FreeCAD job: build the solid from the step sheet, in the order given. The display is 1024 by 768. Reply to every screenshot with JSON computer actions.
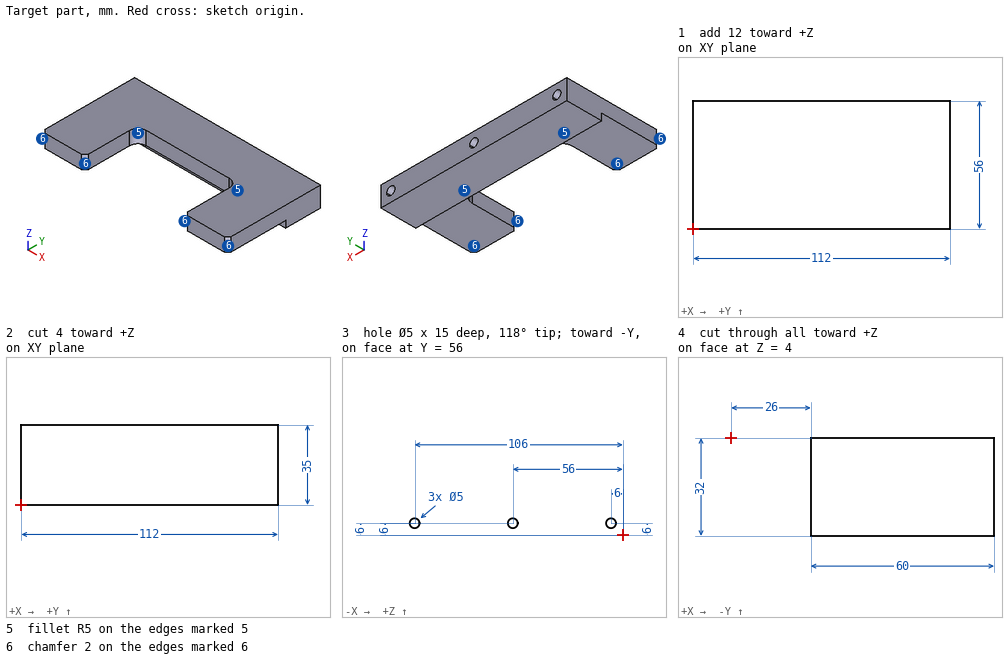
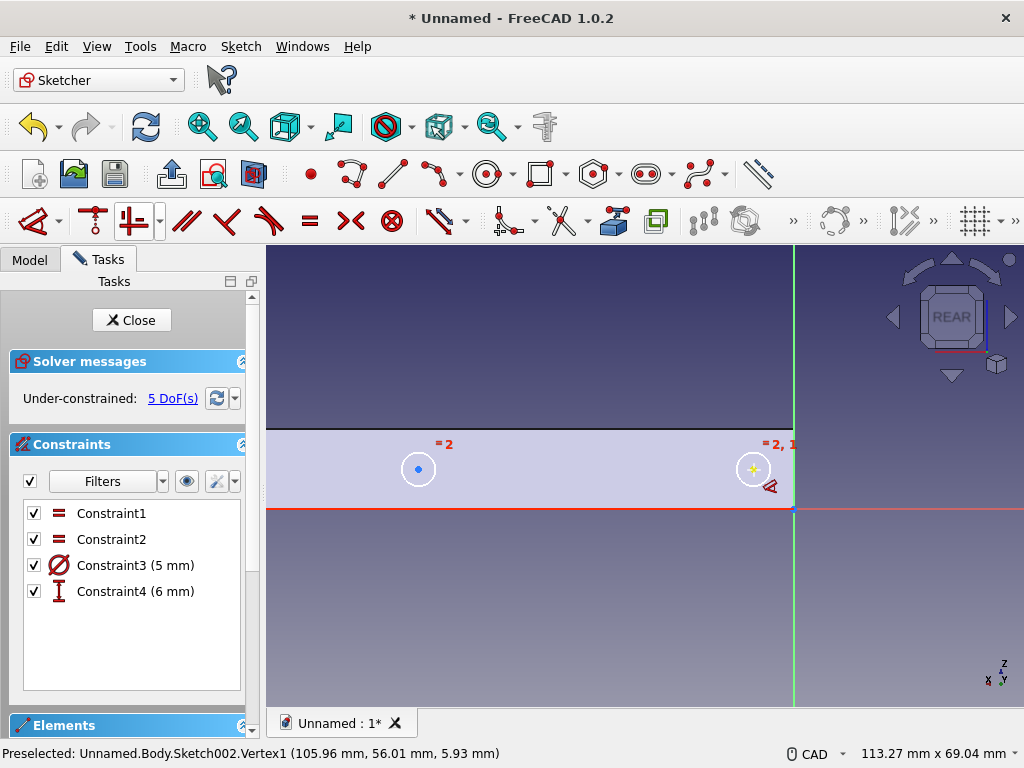
{"action": "left_click", "coordinate": [754, 469]}
{"action": "left_click", "coordinate": [774, 543]}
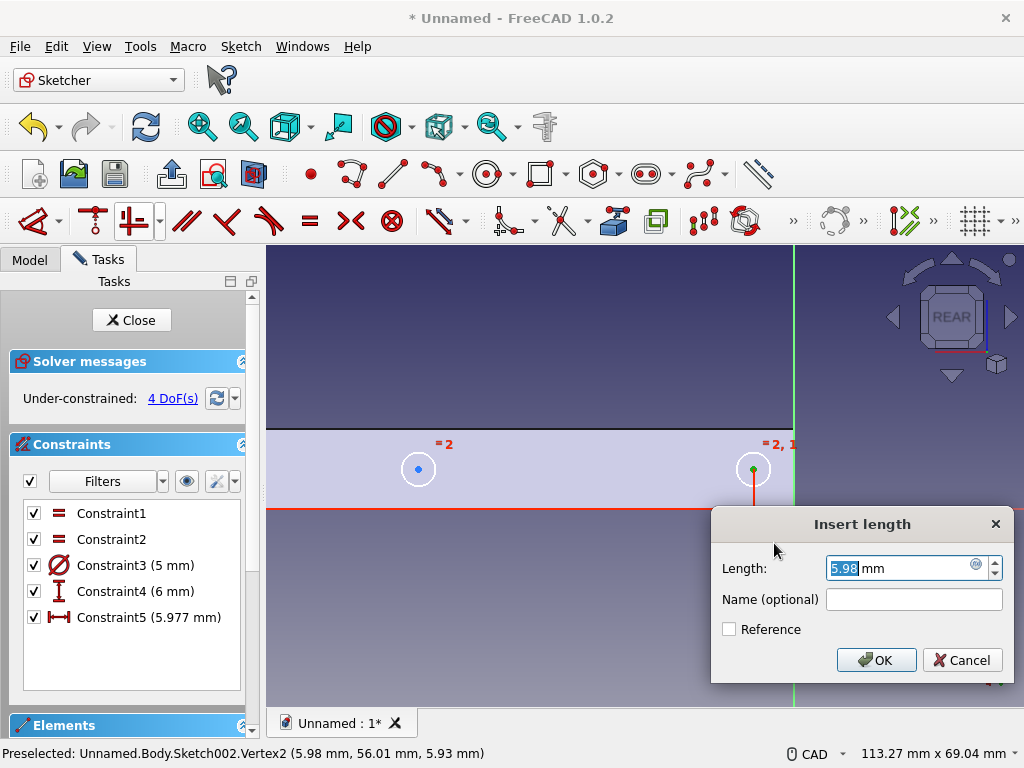
{"action": "type", "text": "6"}
{"action": "key", "text": "Return"}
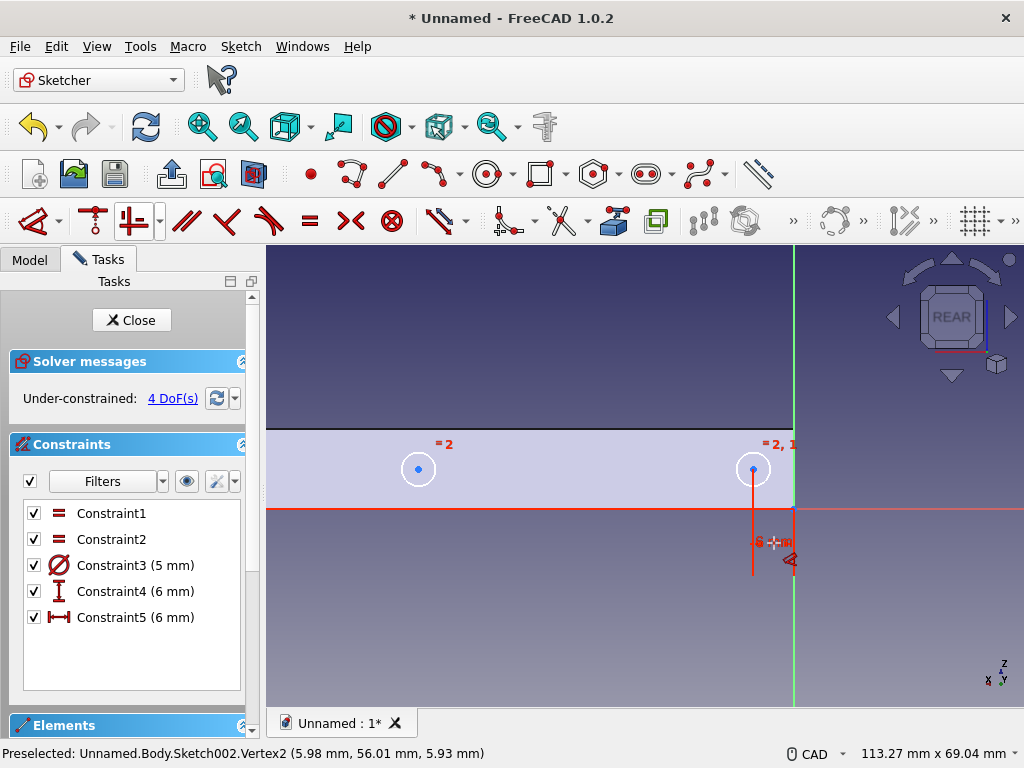
{"action": "left_click", "coordinate": [753, 469]}
{"action": "left_click", "coordinate": [828, 489]}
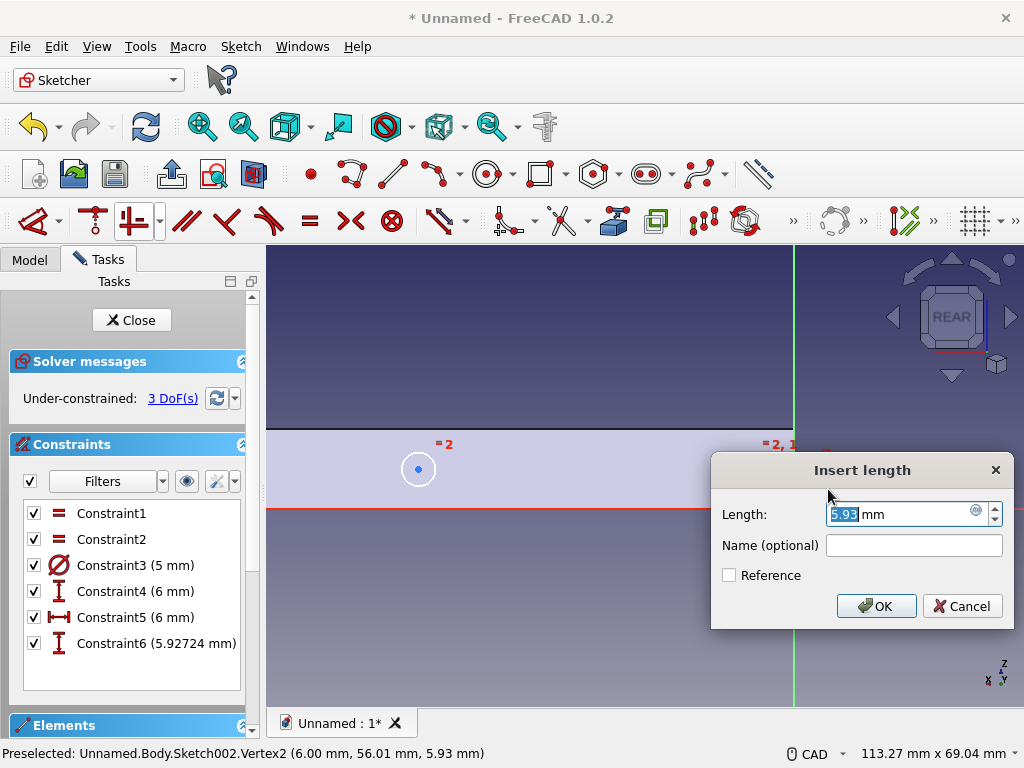
{"action": "type", "text": "6"}
{"action": "key", "text": "Return"}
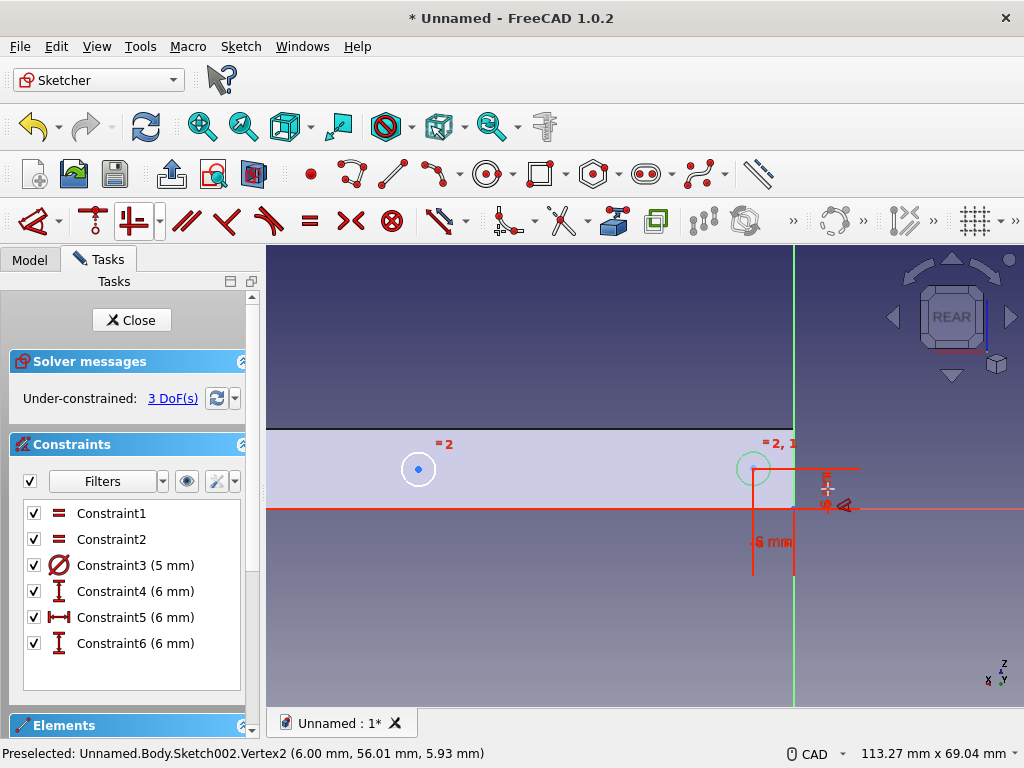
{"action": "left_click", "coordinate": [419, 469]}
{"action": "left_click", "coordinate": [385, 489]}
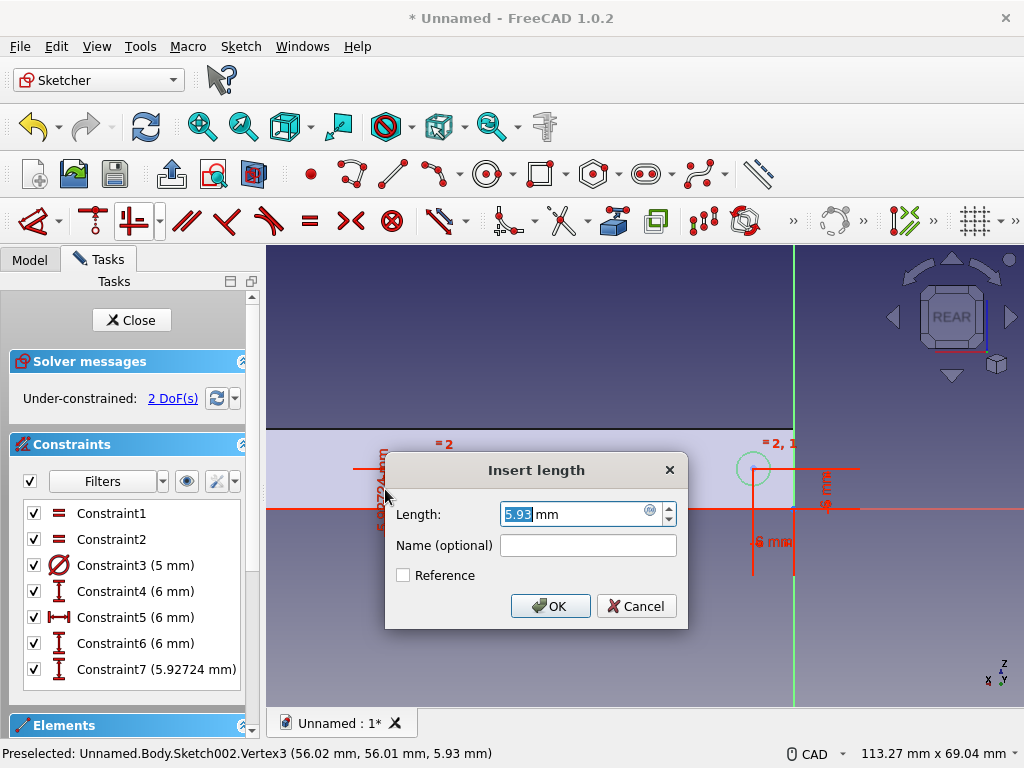
{"action": "type", "text": "6"}
{"action": "key", "text": "Return"}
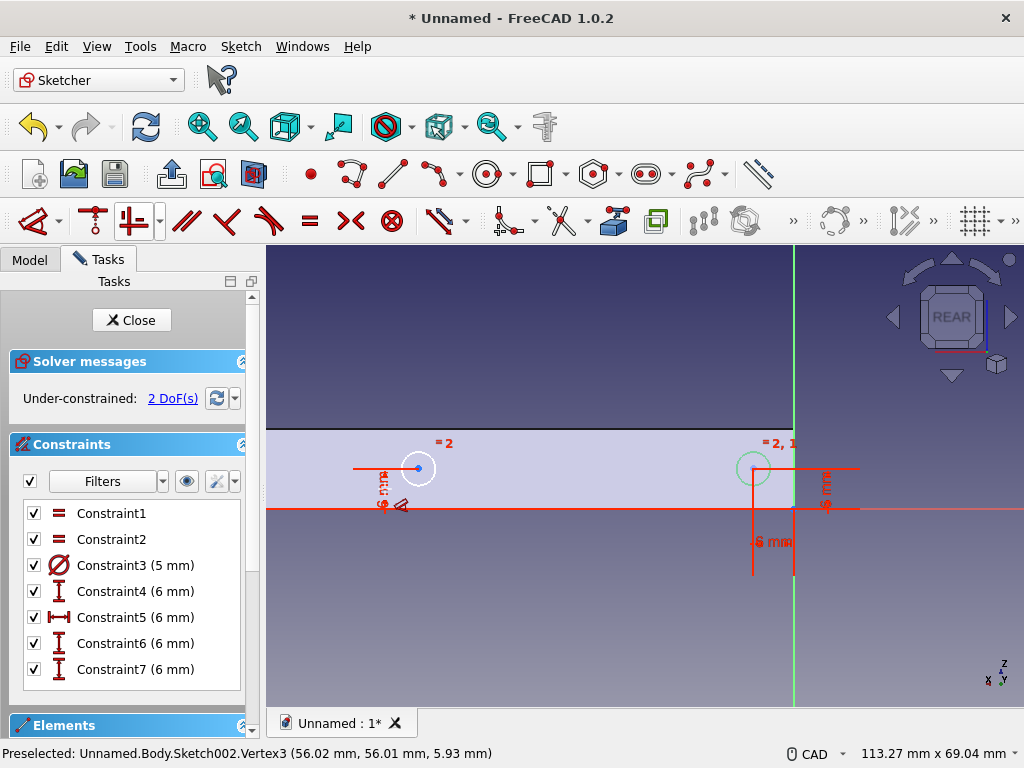
{"action": "left_click", "coordinate": [419, 469]}
{"action": "left_click", "coordinate": [606, 543]}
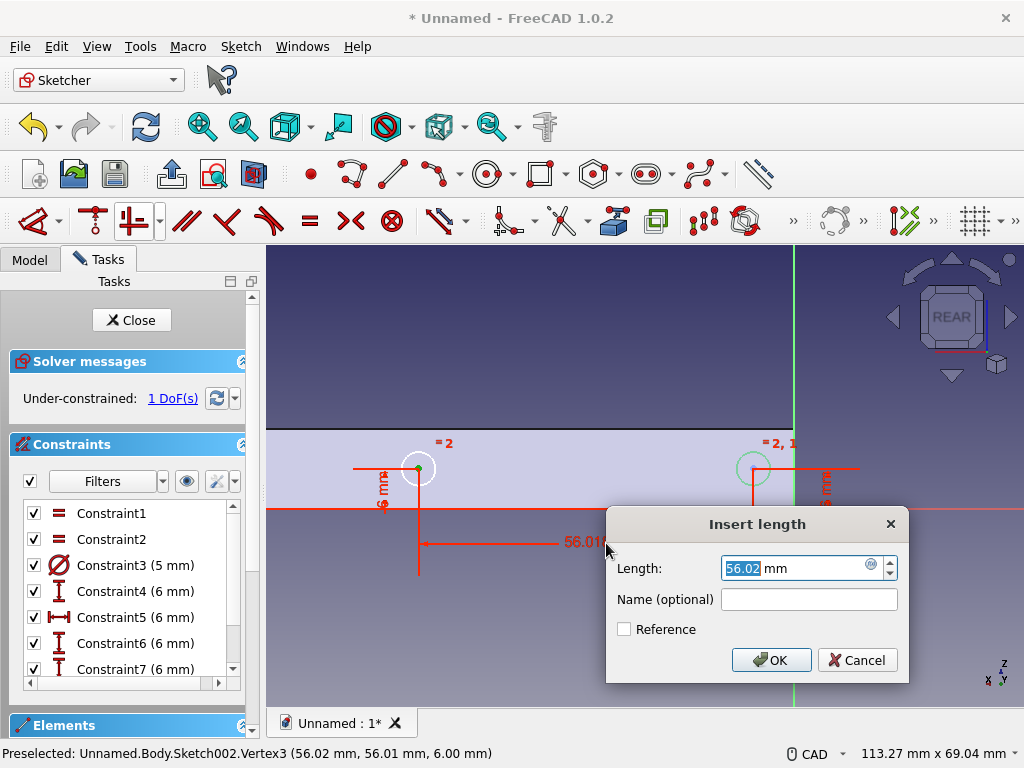
{"action": "type", "text": "56"}
{"action": "key", "text": "Return"}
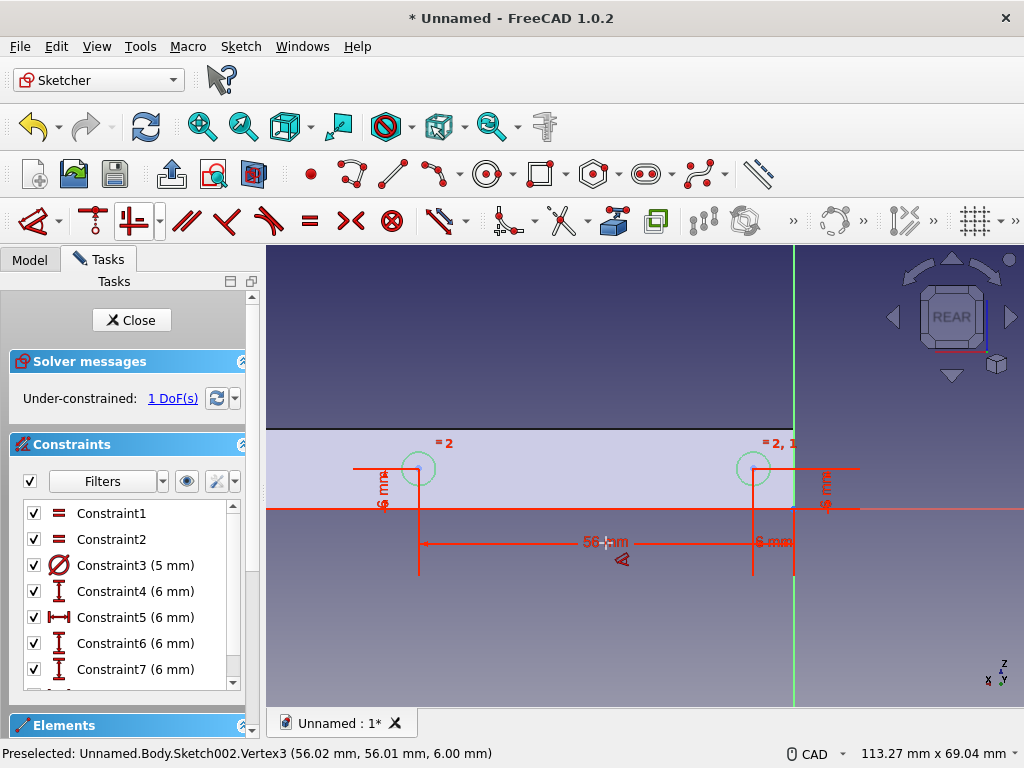
{"action": "scroll", "coordinate": [754, 470], "scroll_direction": "down", "scroll_amount": 3}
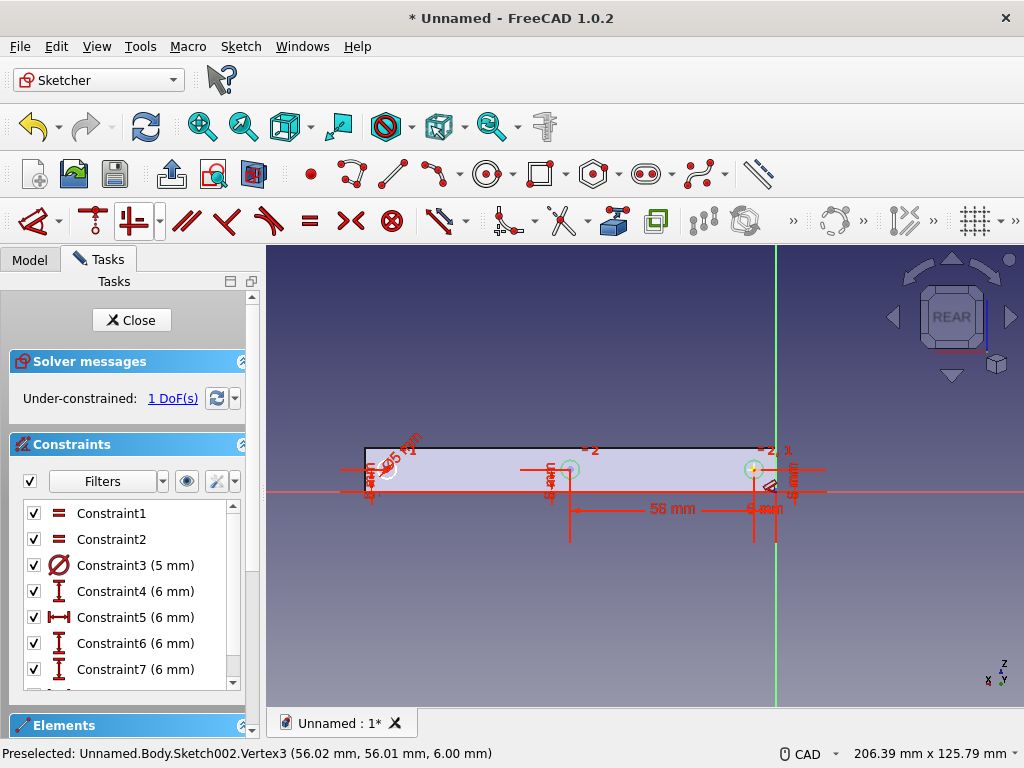
{"action": "left_click", "coordinate": [387, 470]}
{"action": "left_click", "coordinate": [581, 526]}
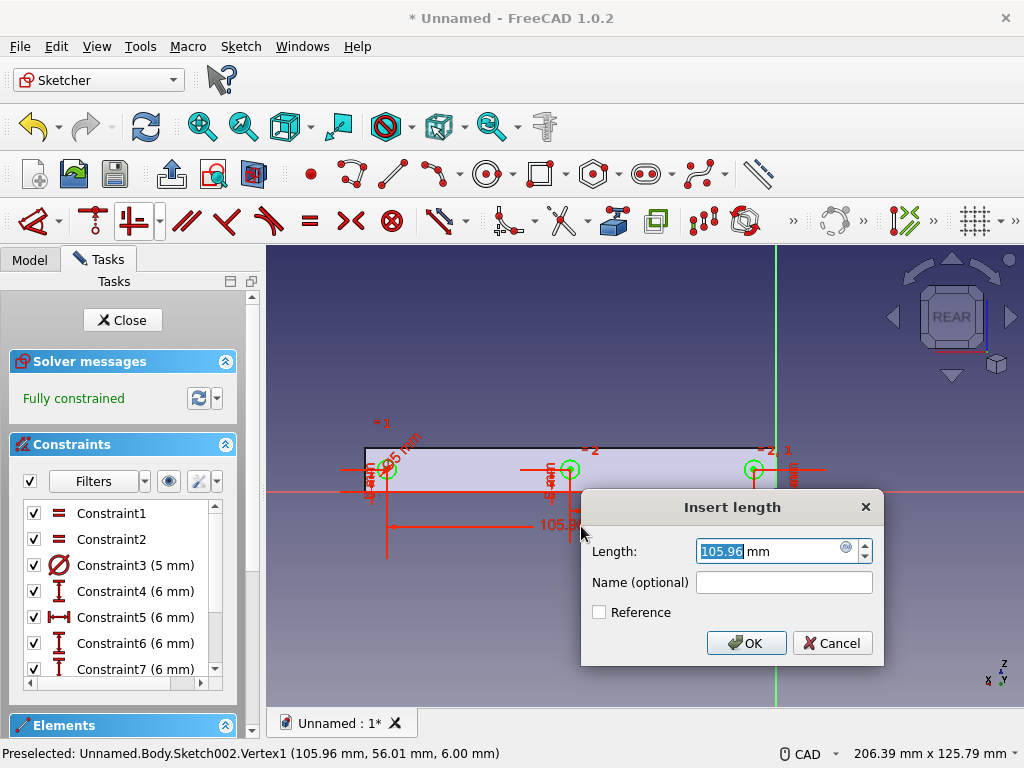
{"action": "type", "text": "106"}
{"action": "key", "text": "Return"}
{"action": "key", "text": "Escape"}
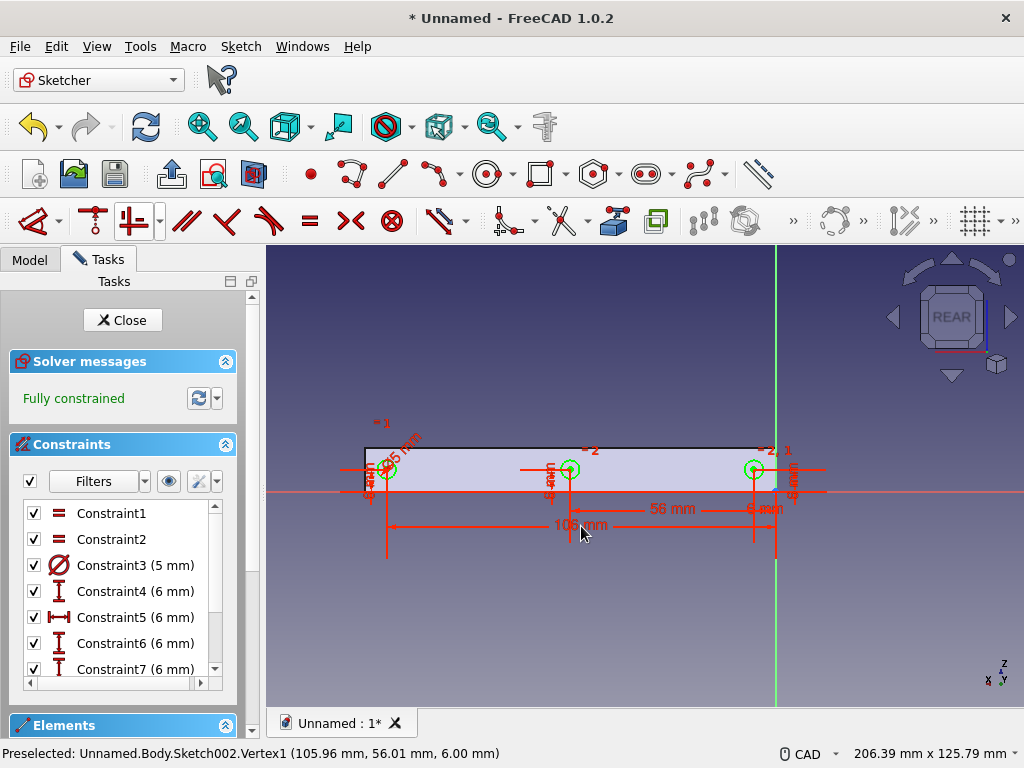
{"action": "left_click", "coordinate": [123, 320]}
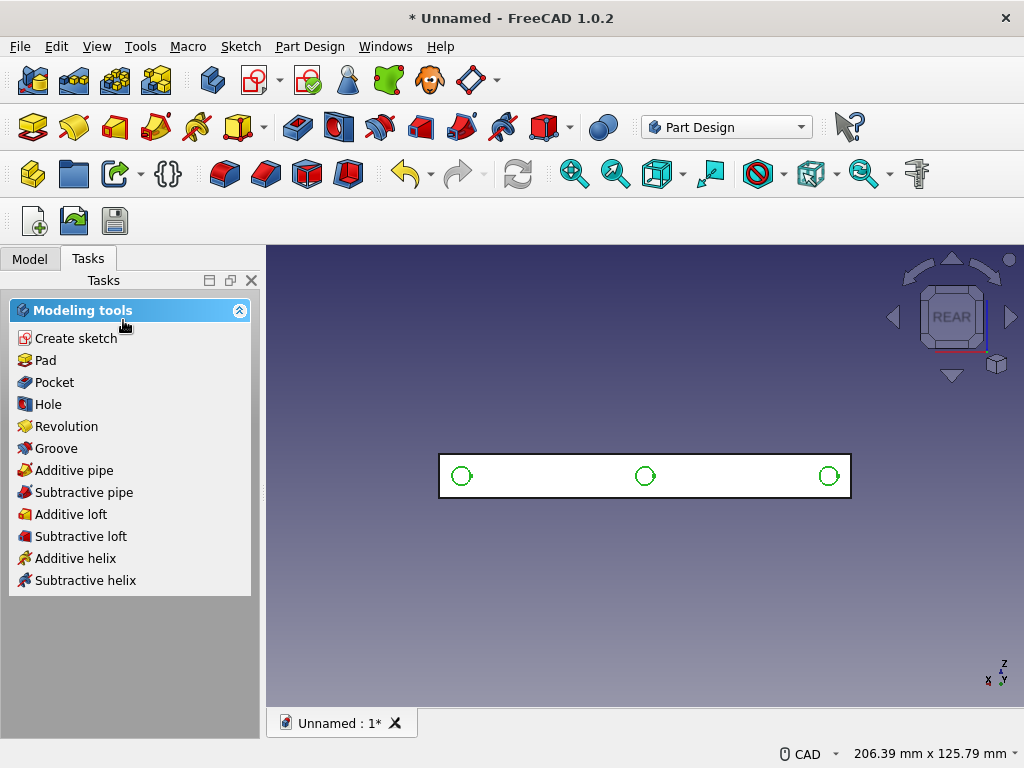
{"action": "left_click", "coordinate": [339, 128]}